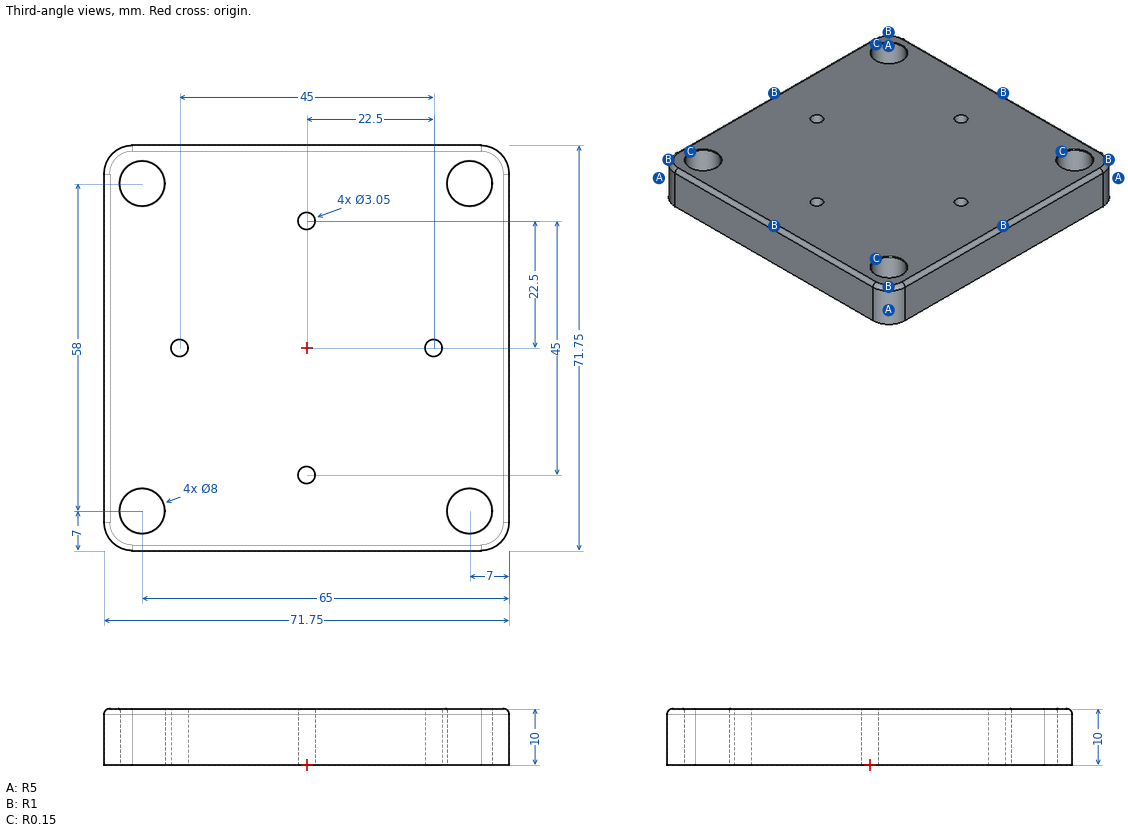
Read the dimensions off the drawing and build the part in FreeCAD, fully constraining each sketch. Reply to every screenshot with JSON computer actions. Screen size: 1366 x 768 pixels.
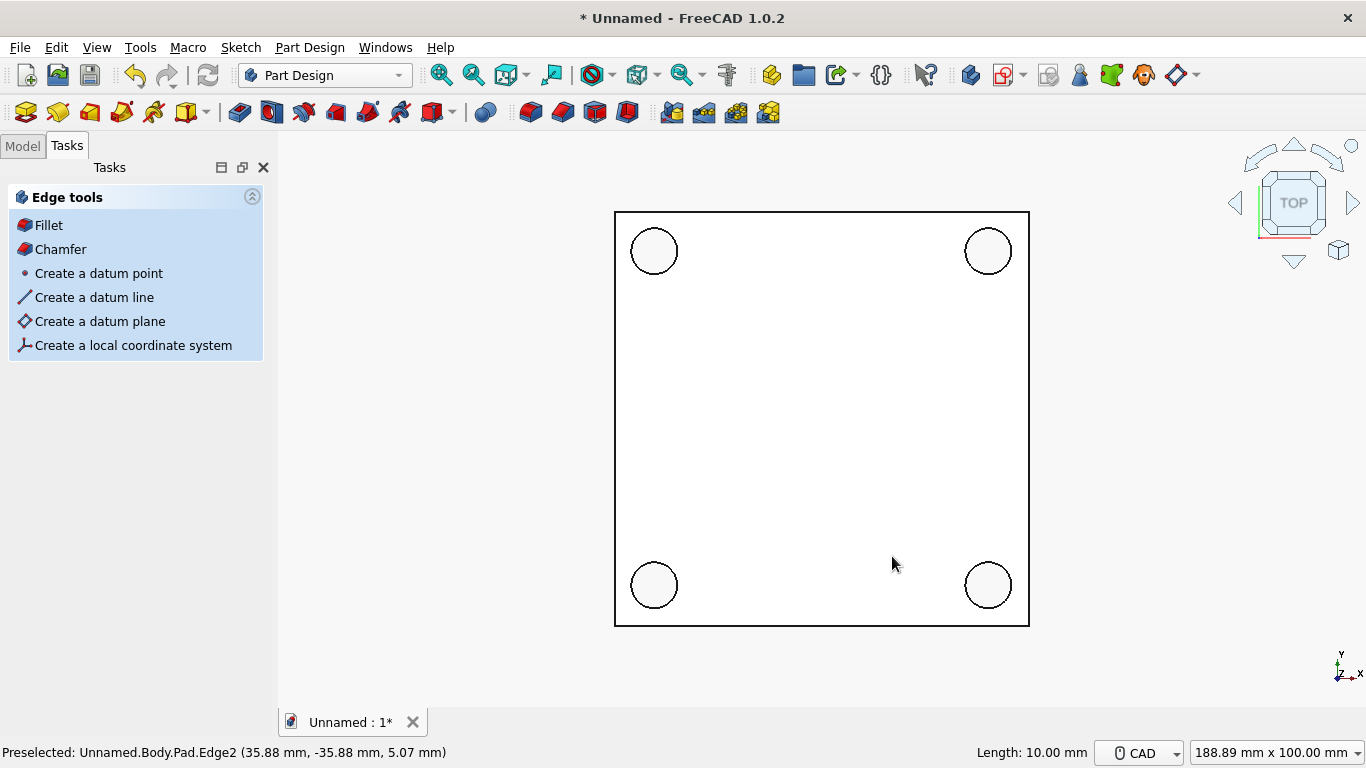
{"action": "key", "text": "1"}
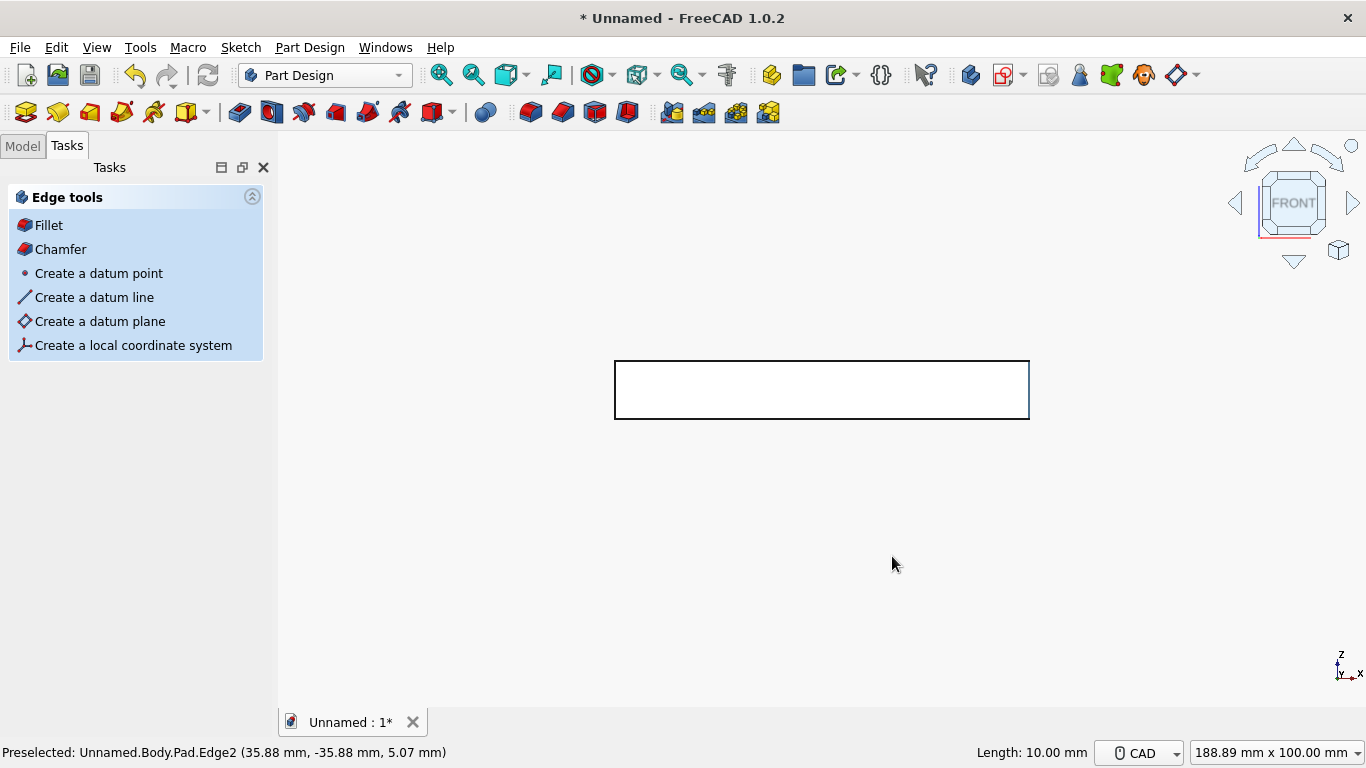
{"action": "left_click", "coordinate": [442, 76]}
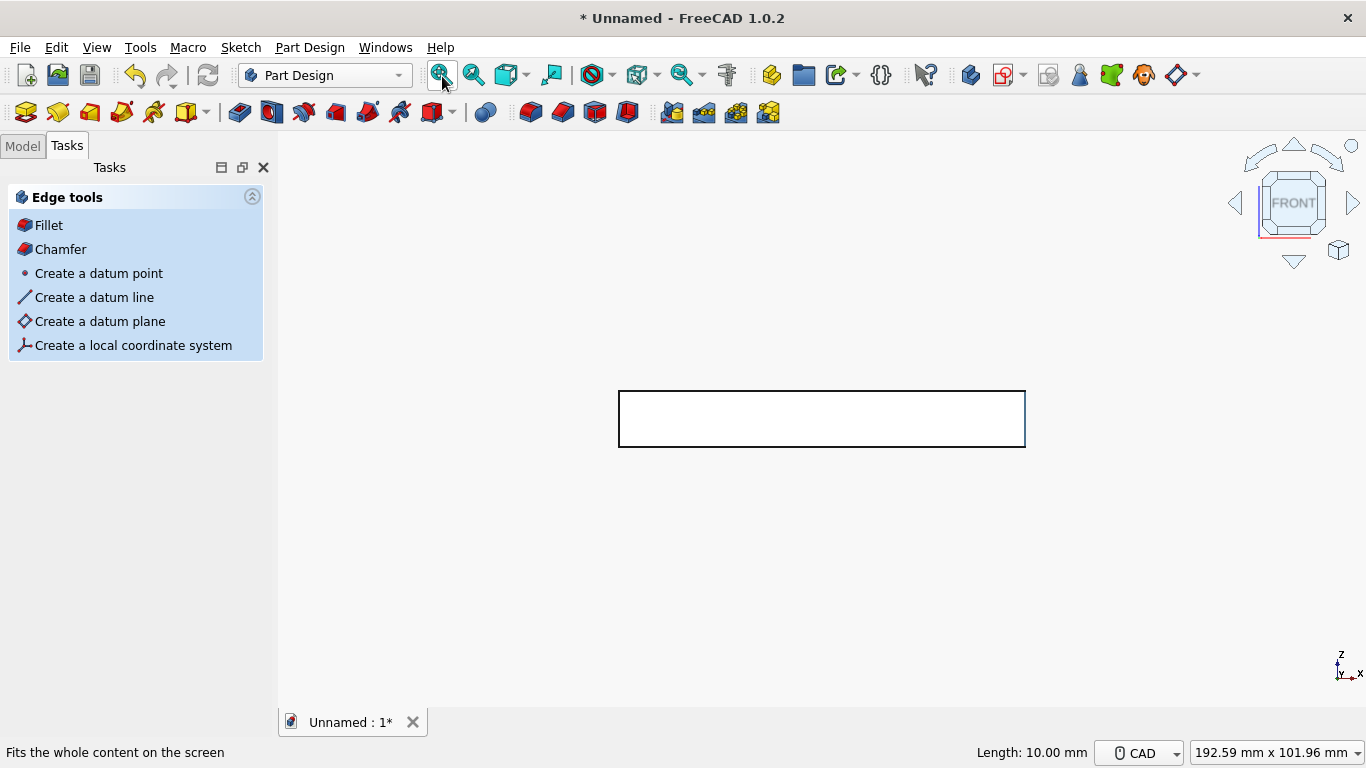
{"action": "left_click", "coordinate": [619, 418], "text": "ctrl"}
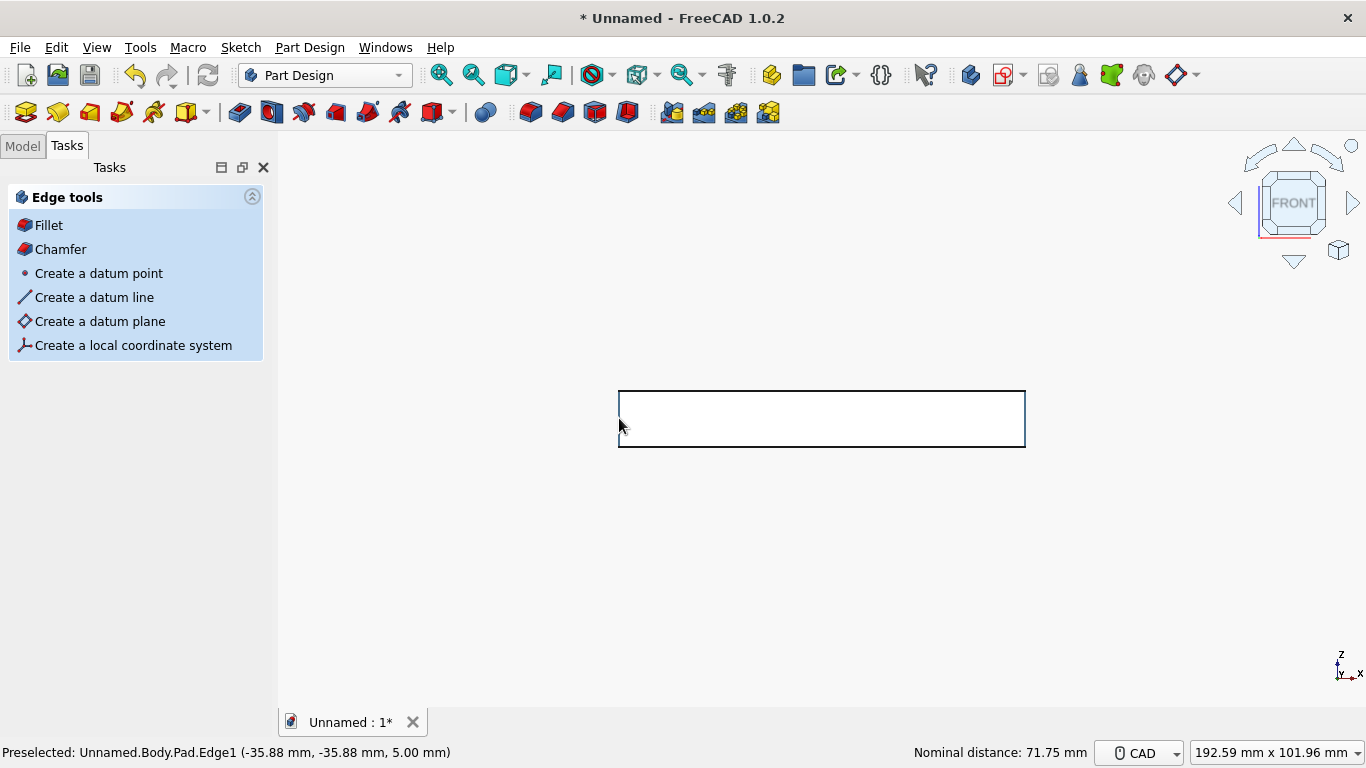
{"action": "key", "text": "3"}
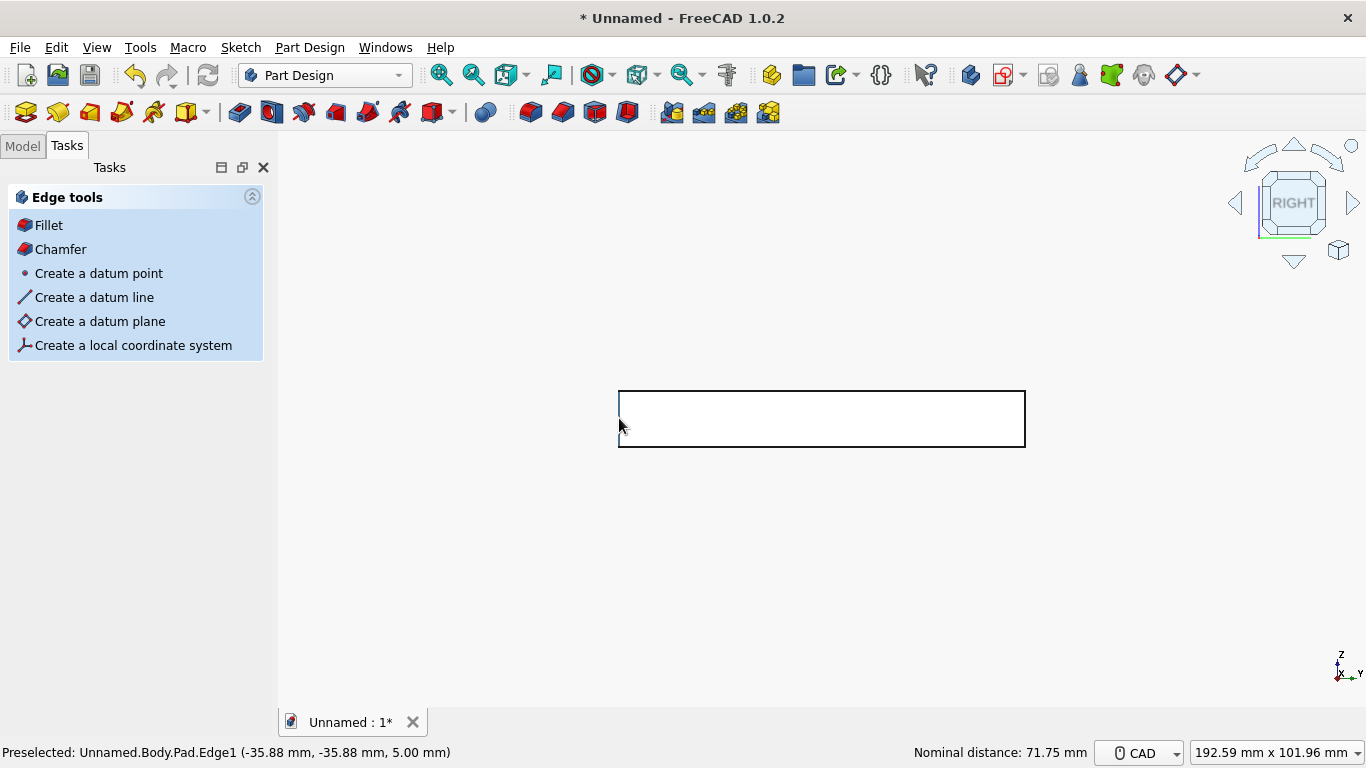
{"action": "left_click", "coordinate": [442, 76]}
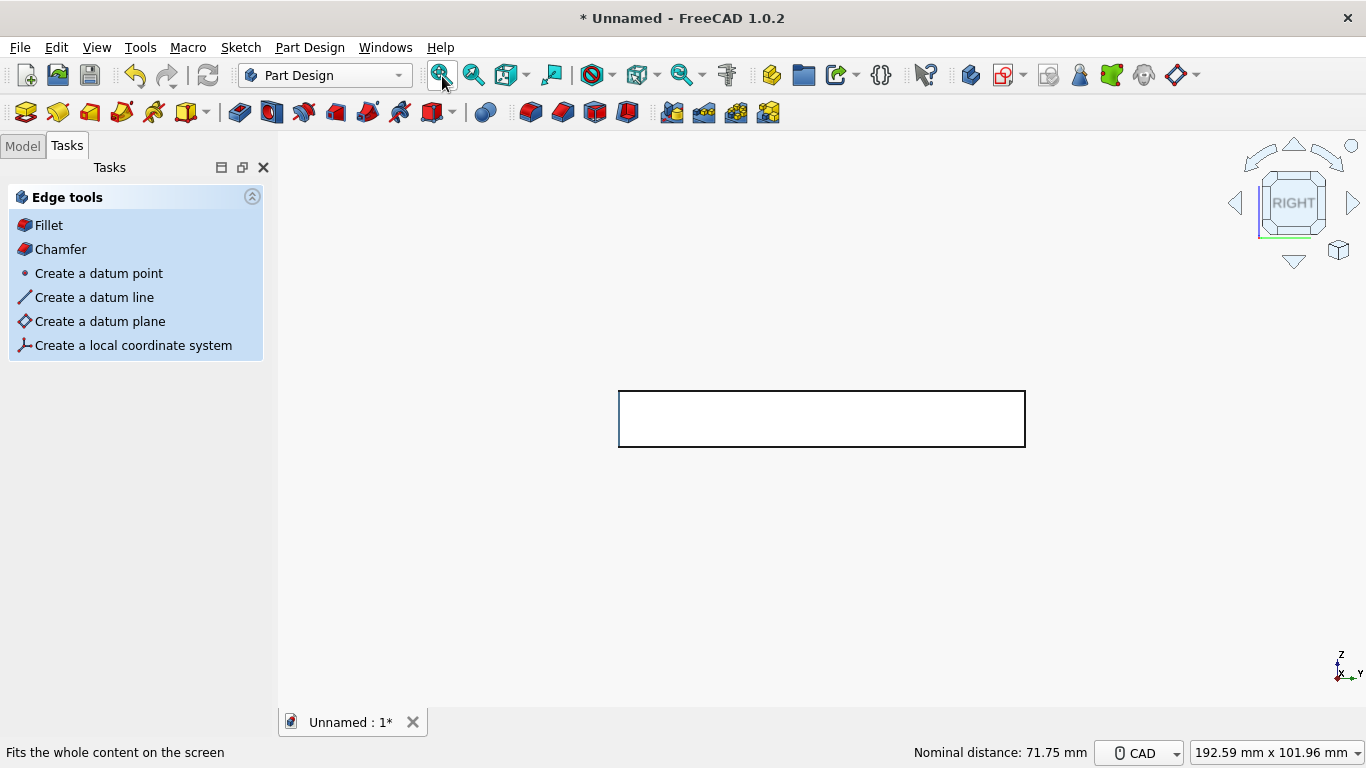
{"action": "left_click", "coordinate": [1025, 418], "text": "ctrl"}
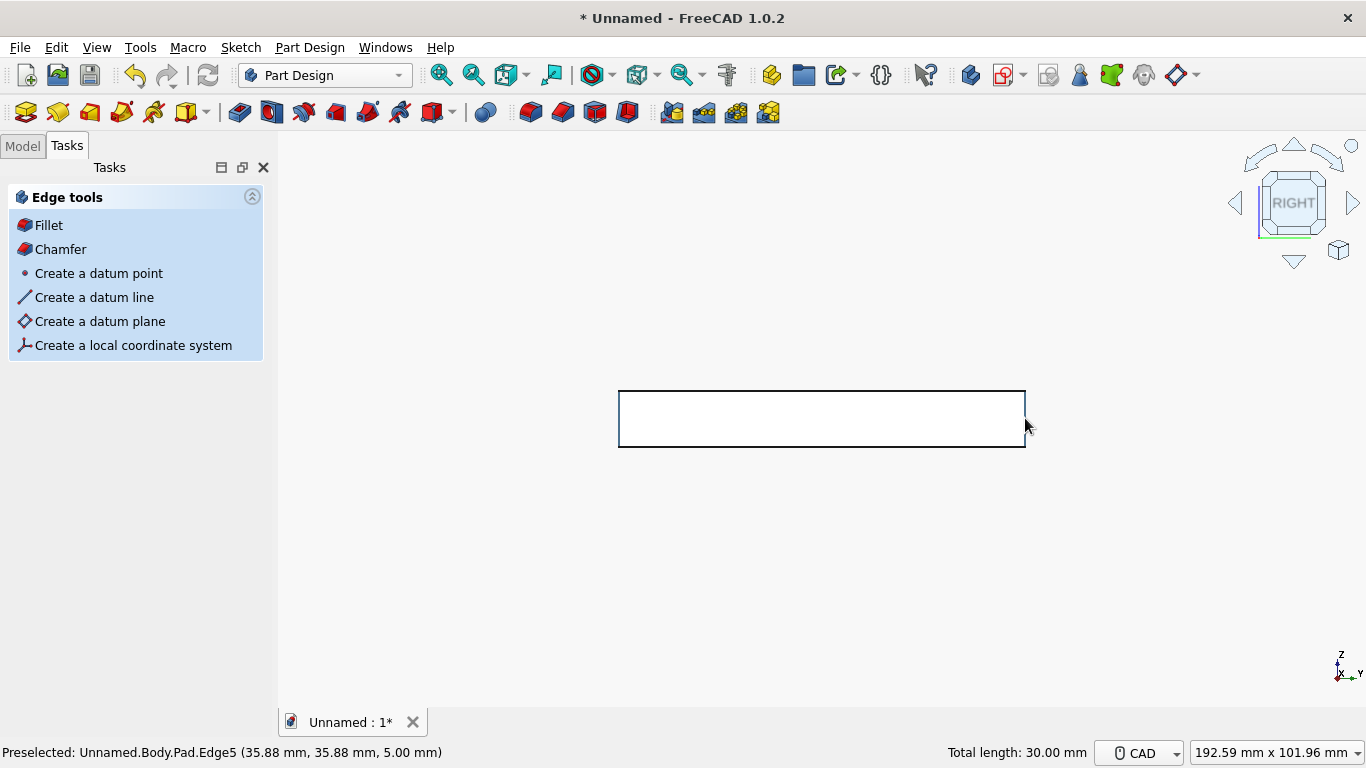
{"action": "key", "text": "5"}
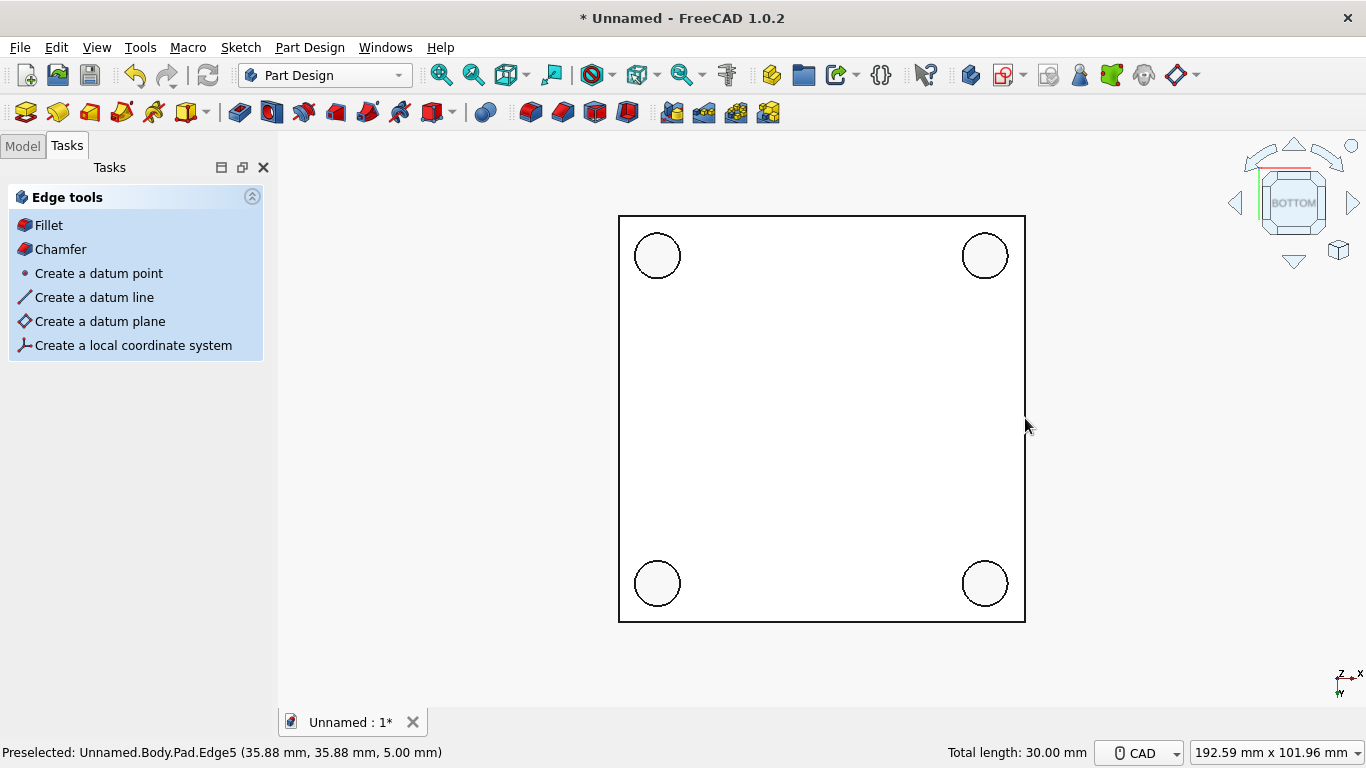
{"action": "key", "text": "4"}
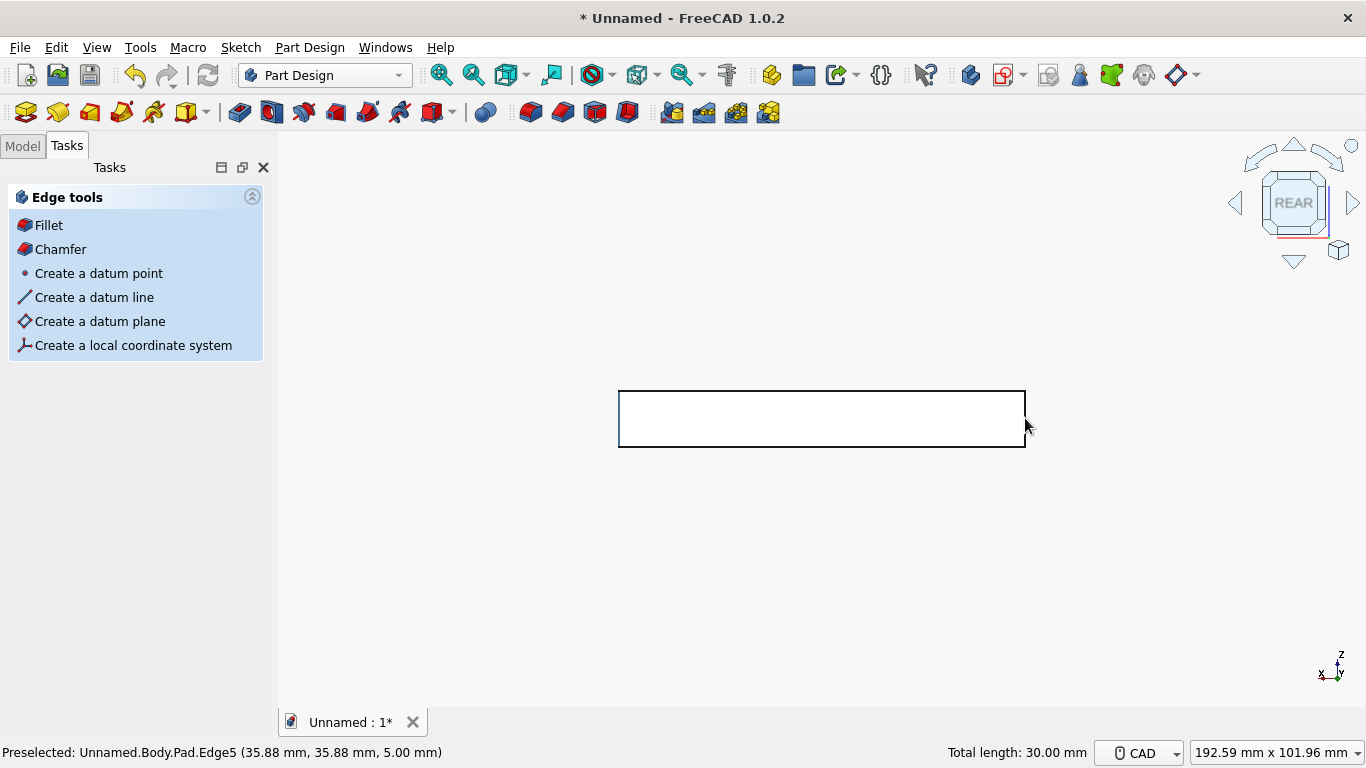
{"action": "left_click", "coordinate": [442, 76]}